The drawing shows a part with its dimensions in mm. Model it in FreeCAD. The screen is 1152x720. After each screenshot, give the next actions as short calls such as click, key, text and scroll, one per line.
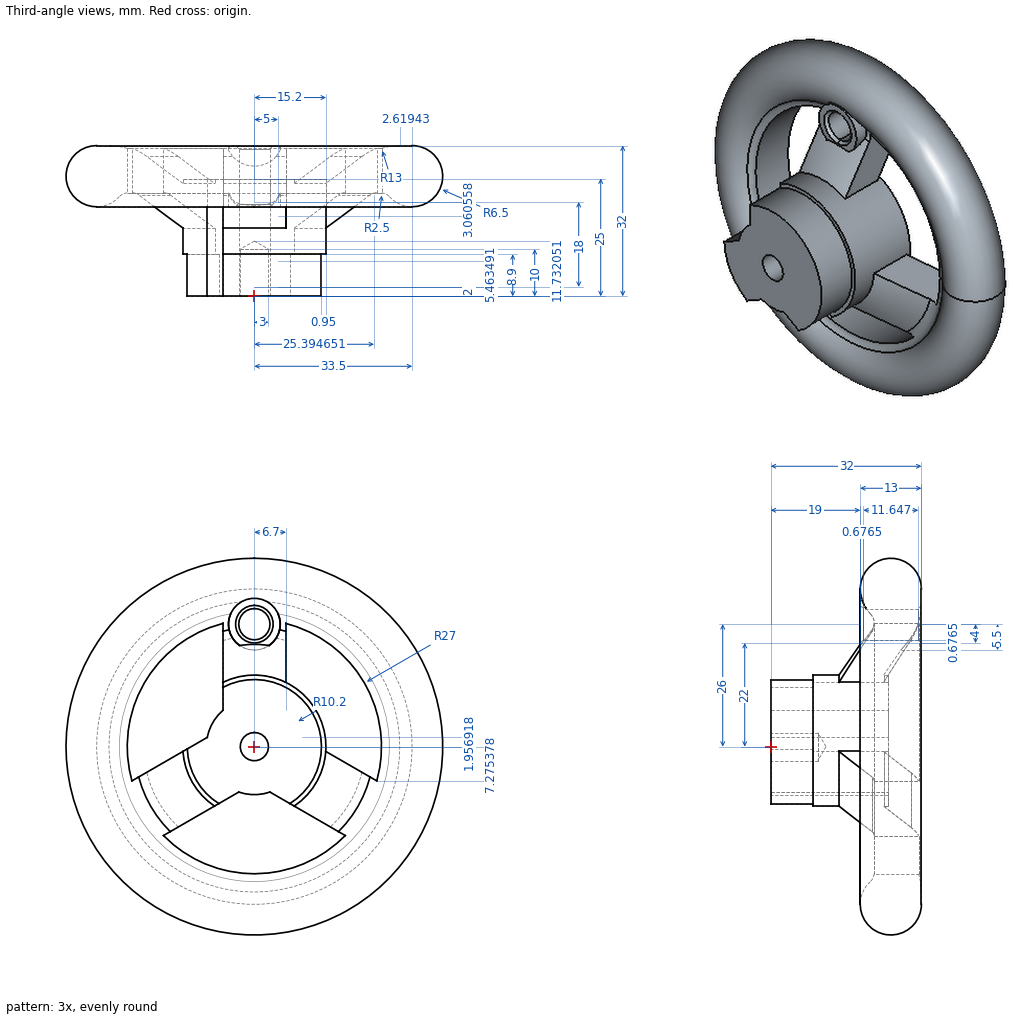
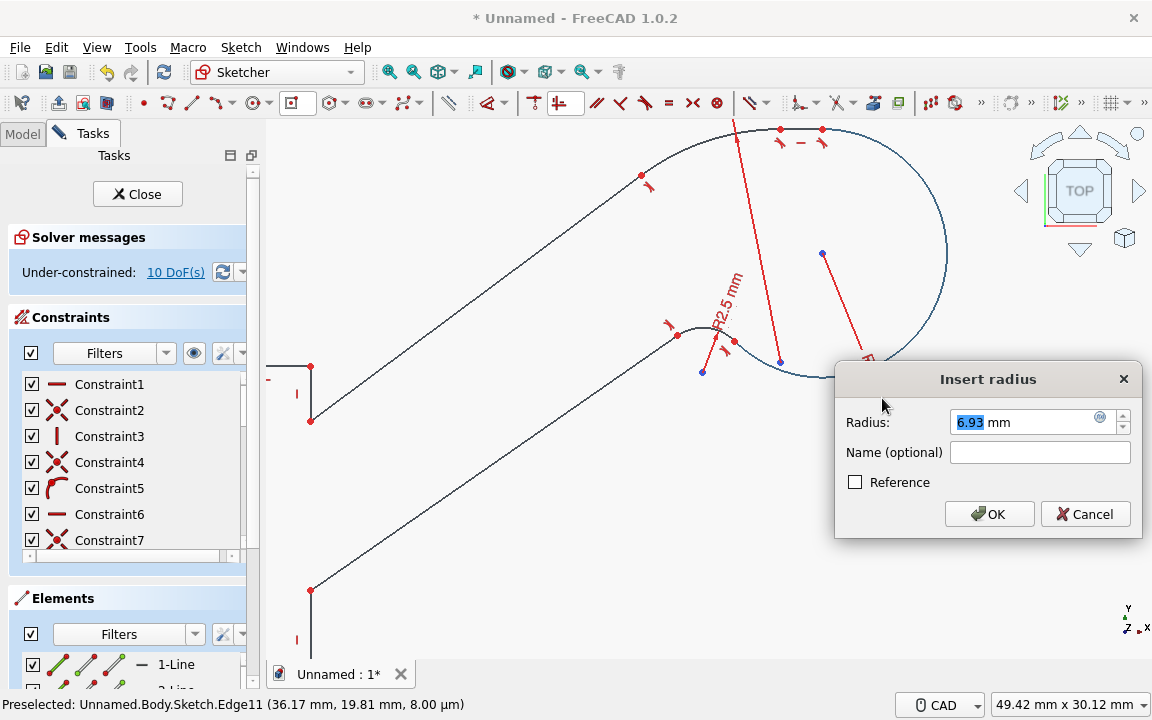
text(6.5)
key(Return)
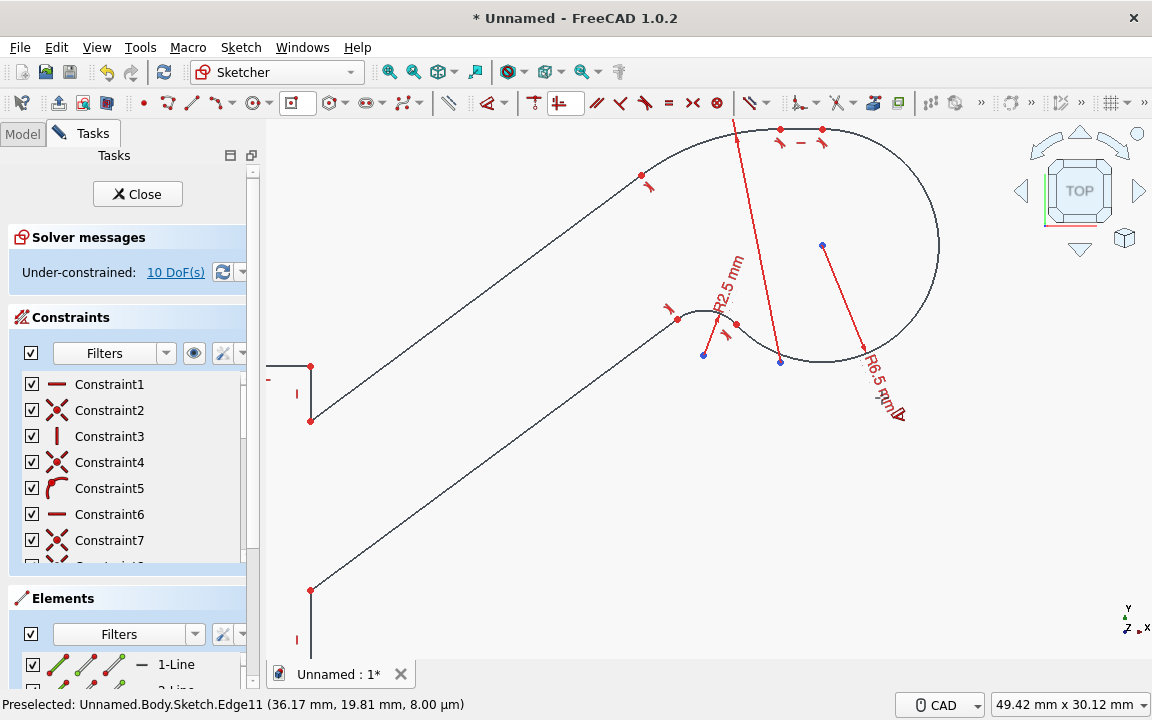
scroll(720, 331, down, 3)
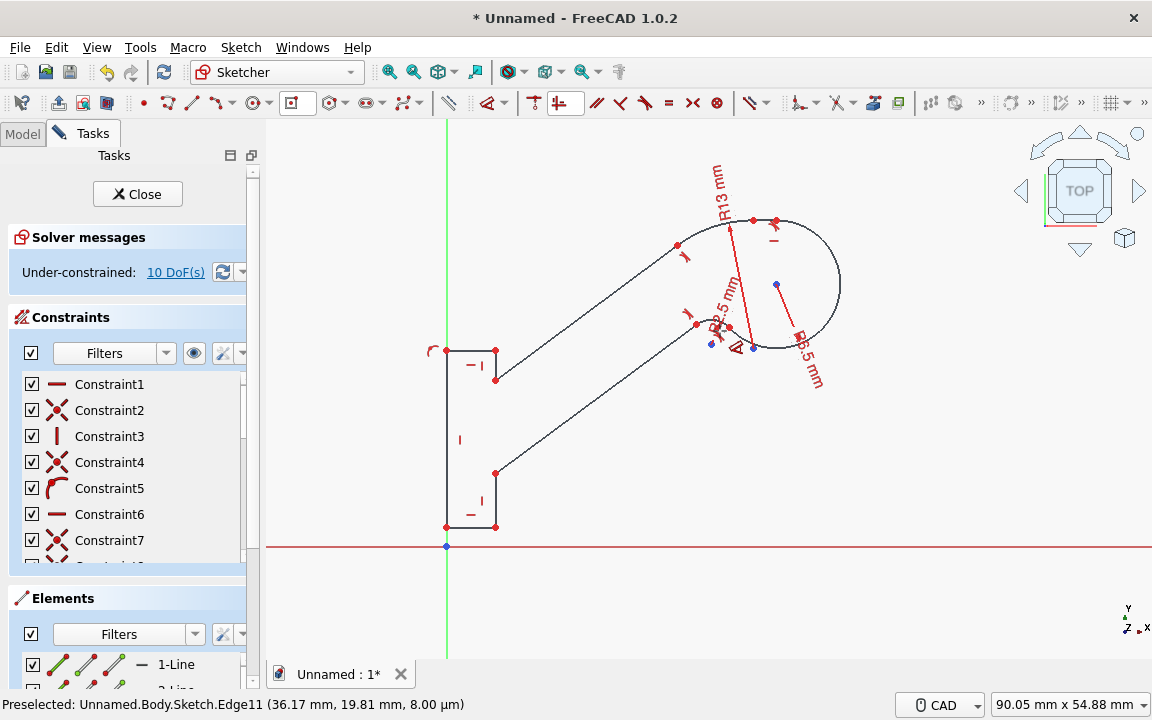
click(481, 351)
click(471, 317)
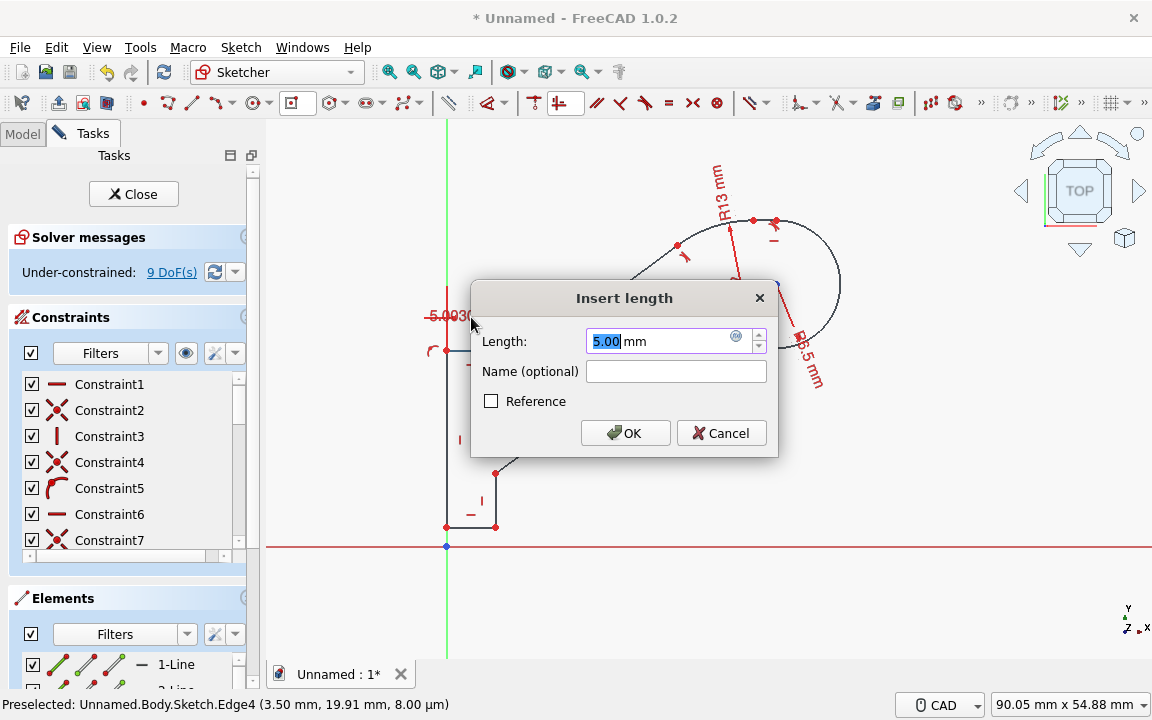
text(5)
key(Return)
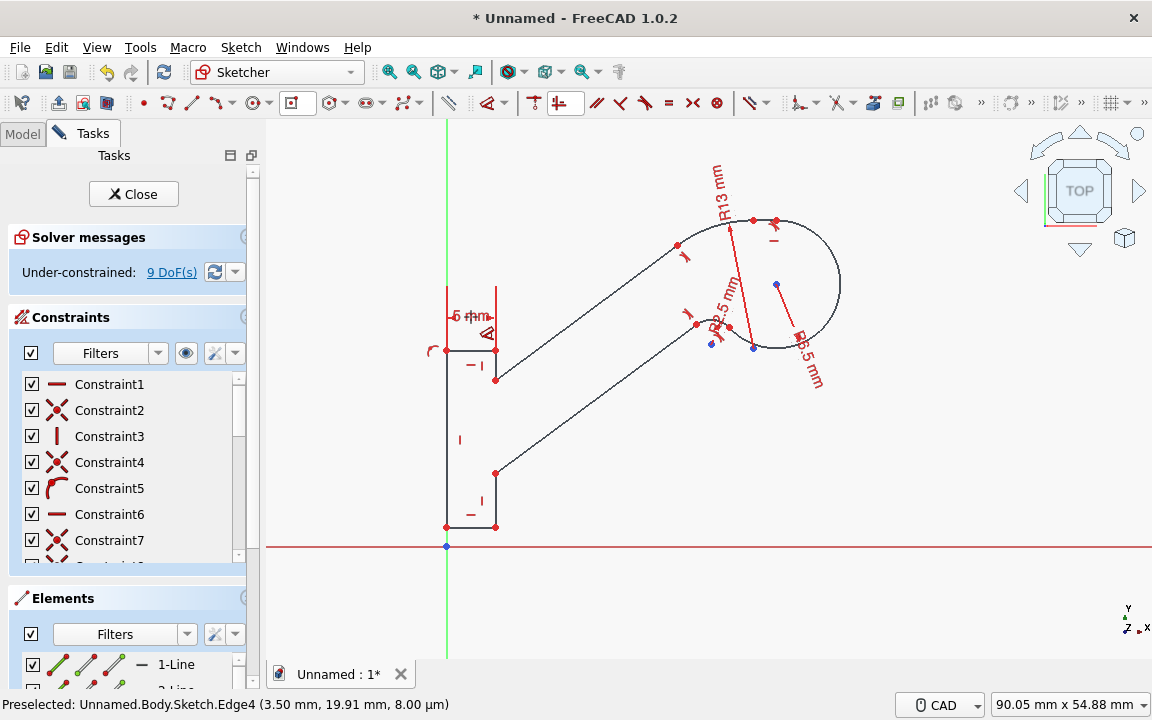
click(461, 528)
click(471, 562)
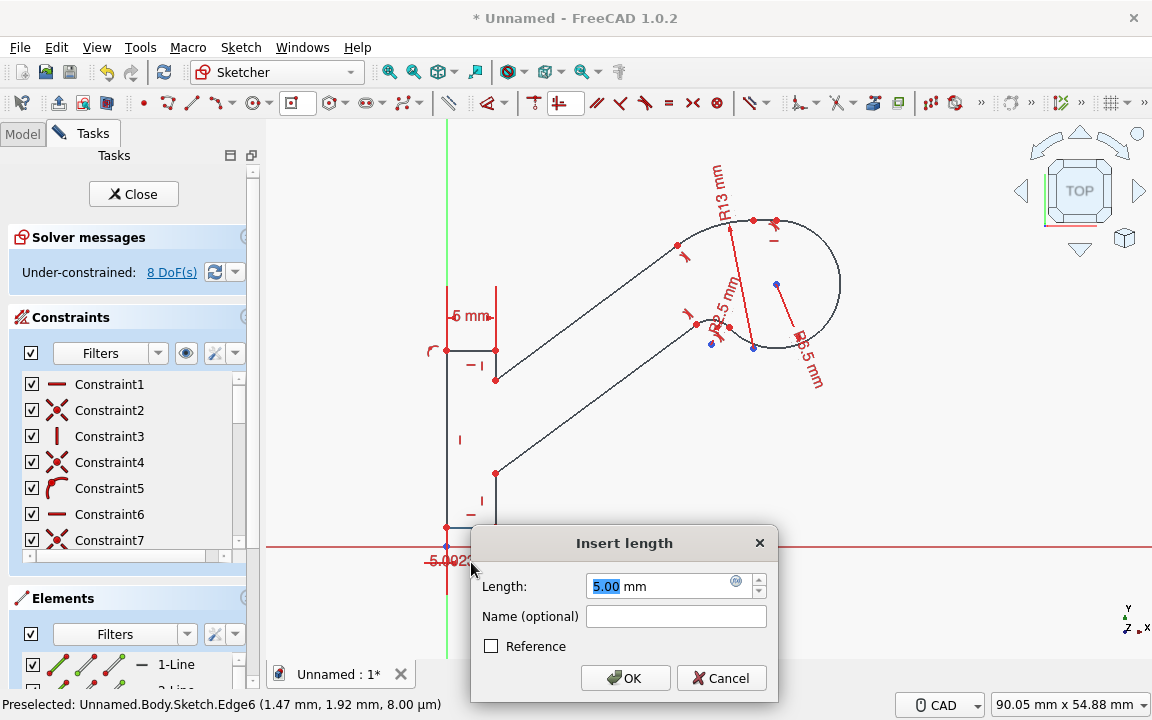
text(5)
key(Return)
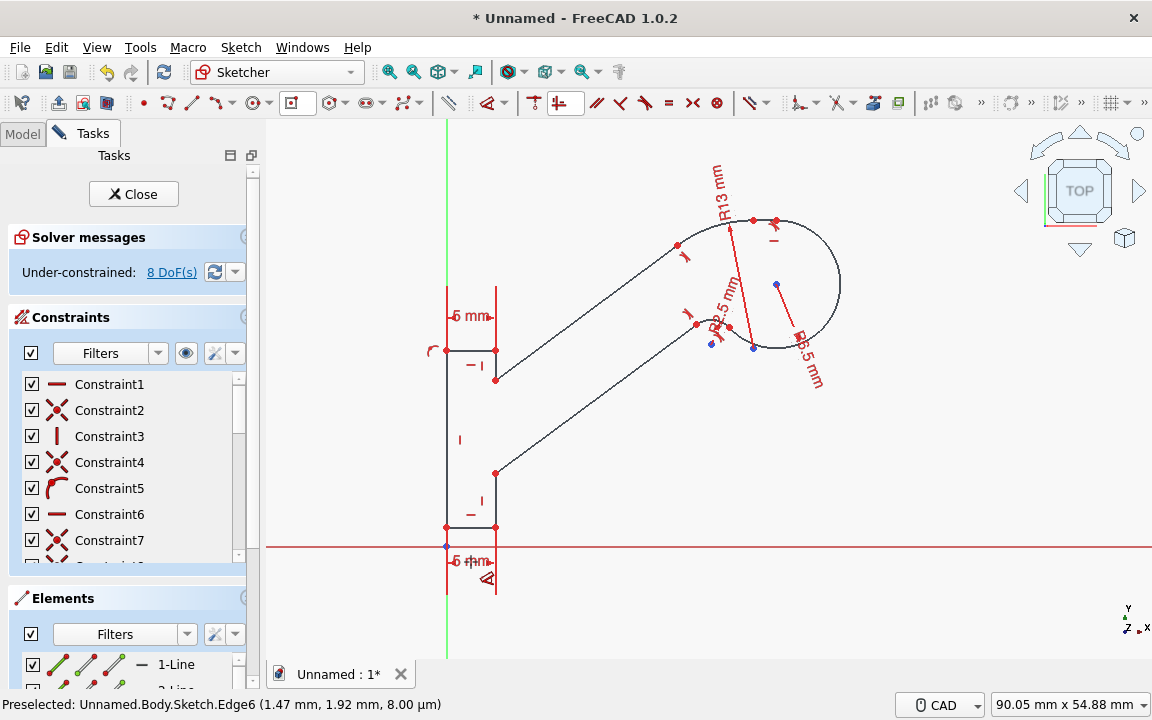
click(447, 404)
click(413, 439)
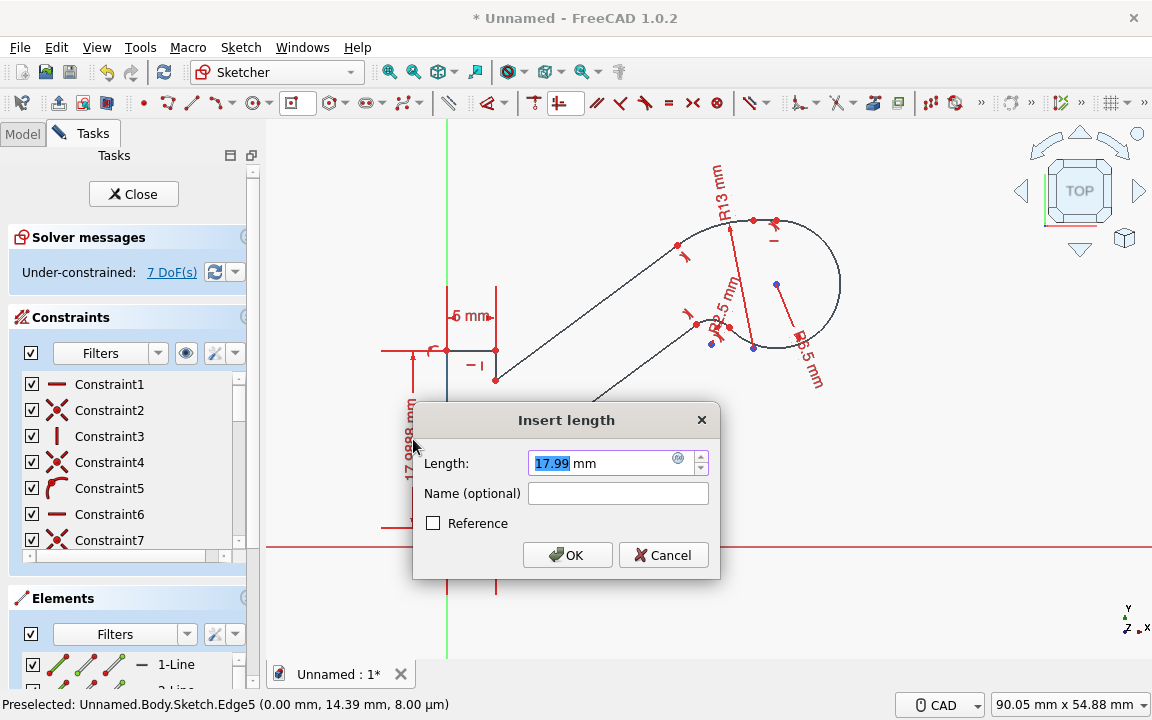
text(18)
key(Return)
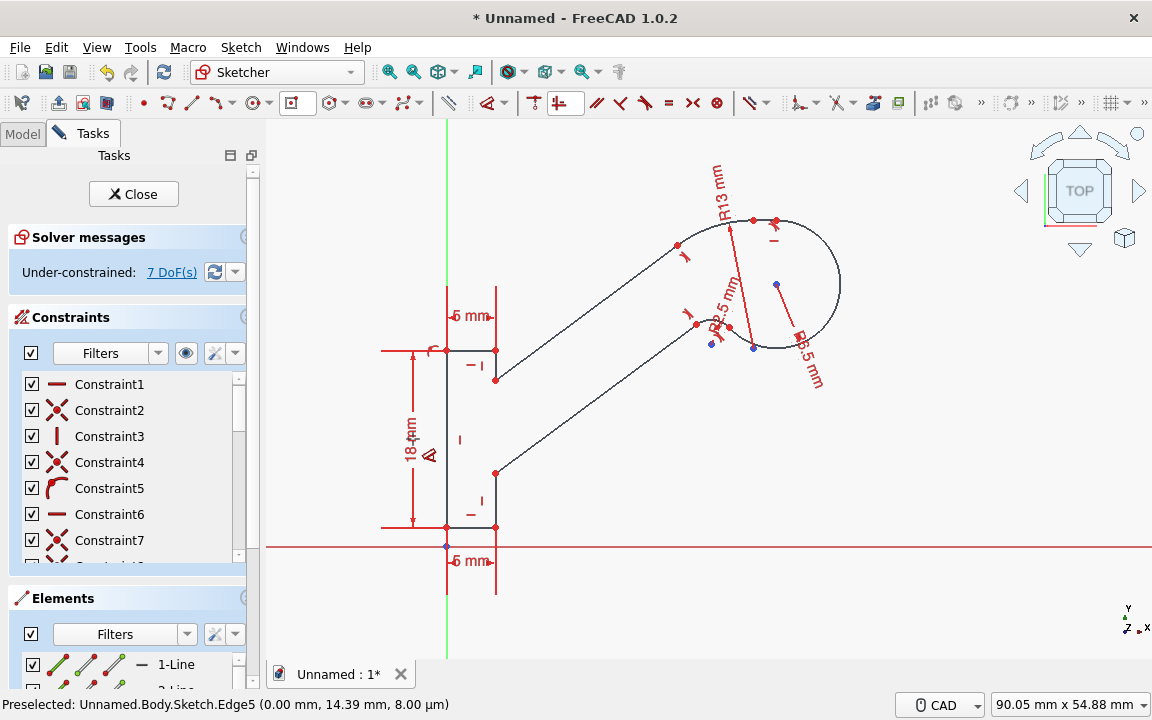
scroll(447, 528, up, 4)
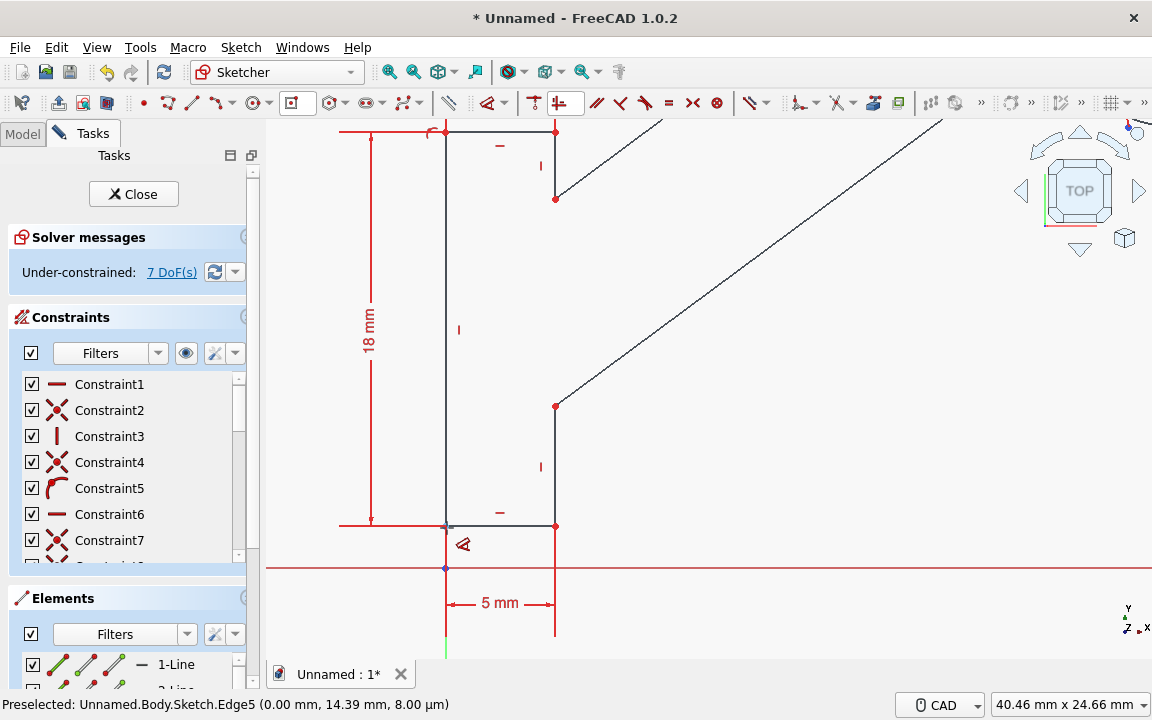
click(446, 526)
click(412, 547)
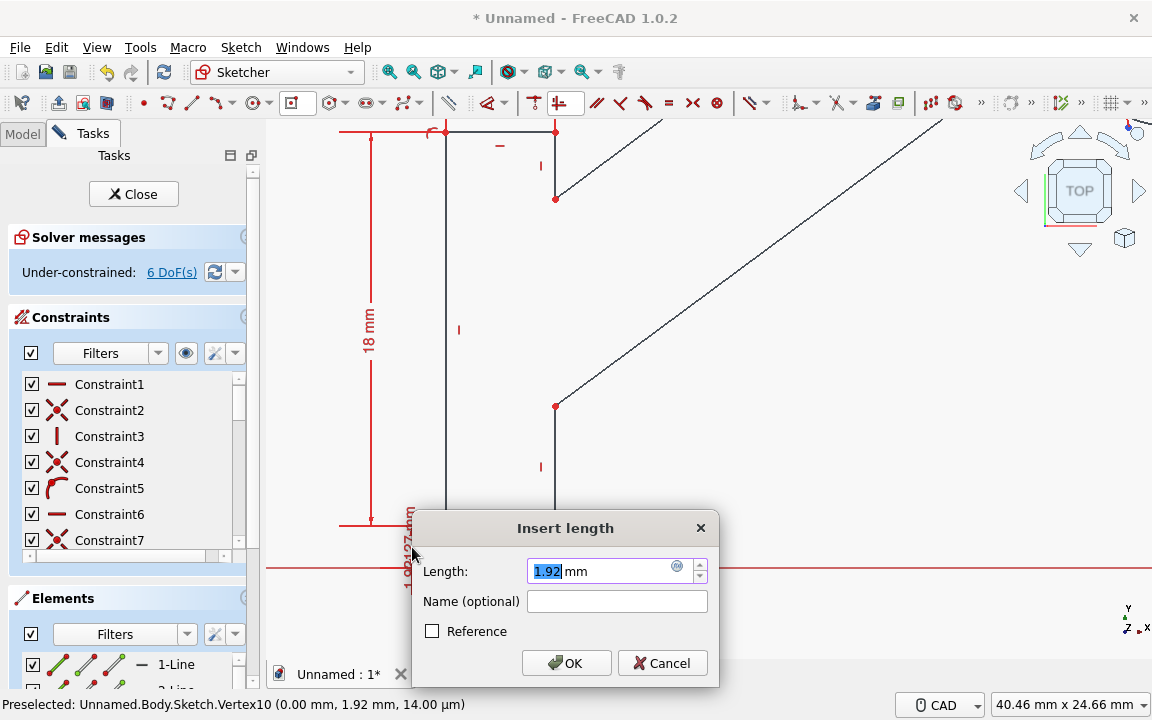
text(2)
key(Return)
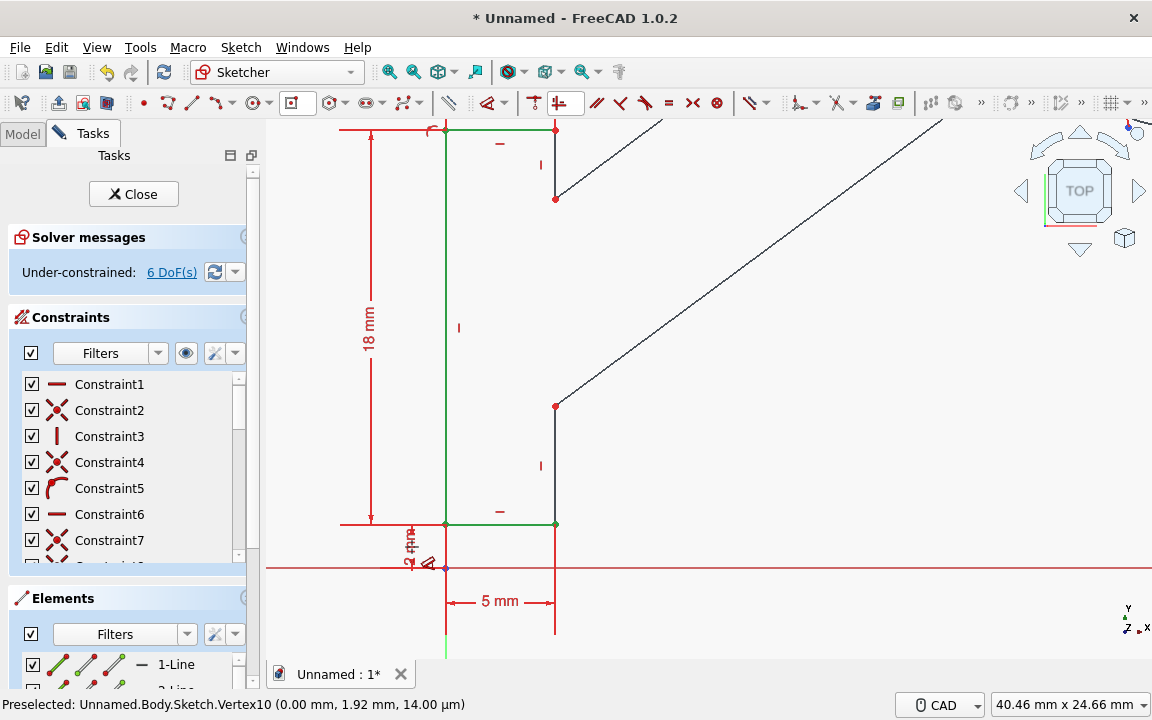
scroll(447, 529, down, 4)